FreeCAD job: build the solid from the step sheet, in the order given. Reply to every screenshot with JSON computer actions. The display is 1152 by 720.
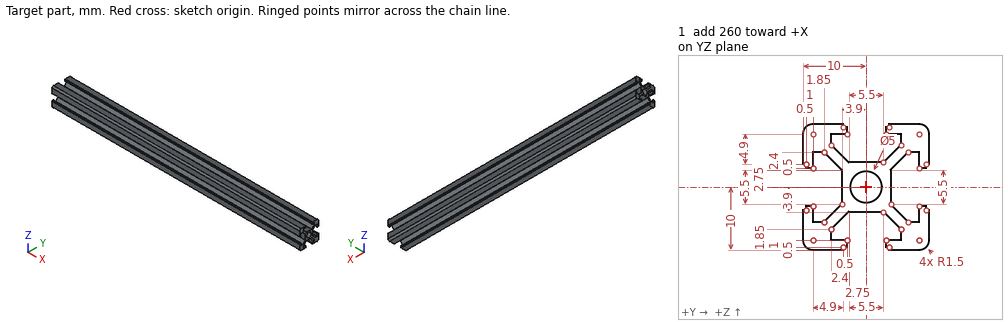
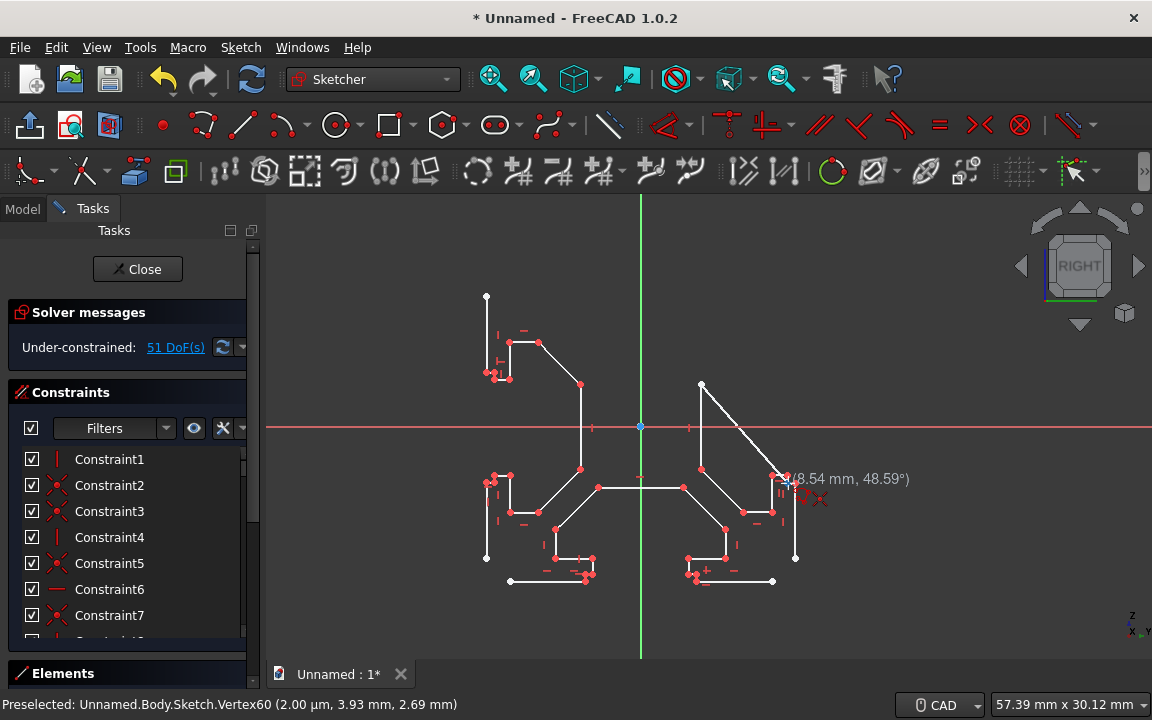
{"action": "left_click", "coordinate": [744, 342]}
{"action": "left_click", "coordinate": [772, 342]}
{"action": "left_click", "coordinate": [772, 379]}
{"action": "left_click", "coordinate": [788, 379]}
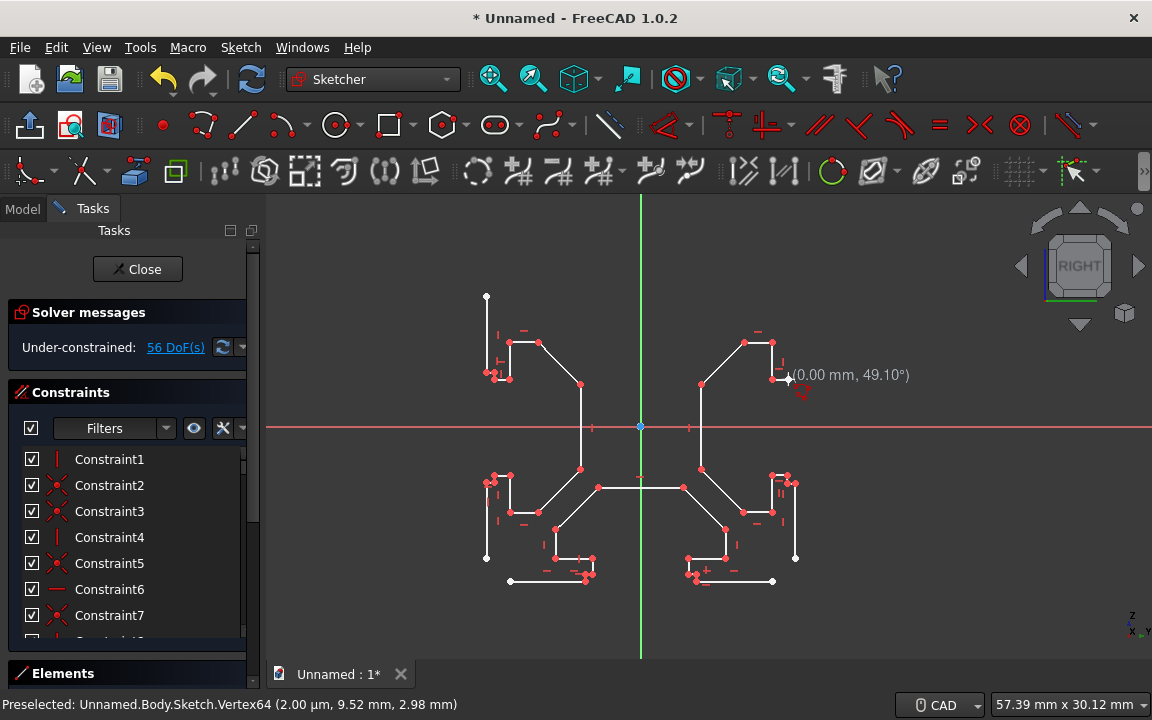
{"action": "scroll", "coordinate": [788, 371], "scroll_direction": "up", "scroll_amount": 4}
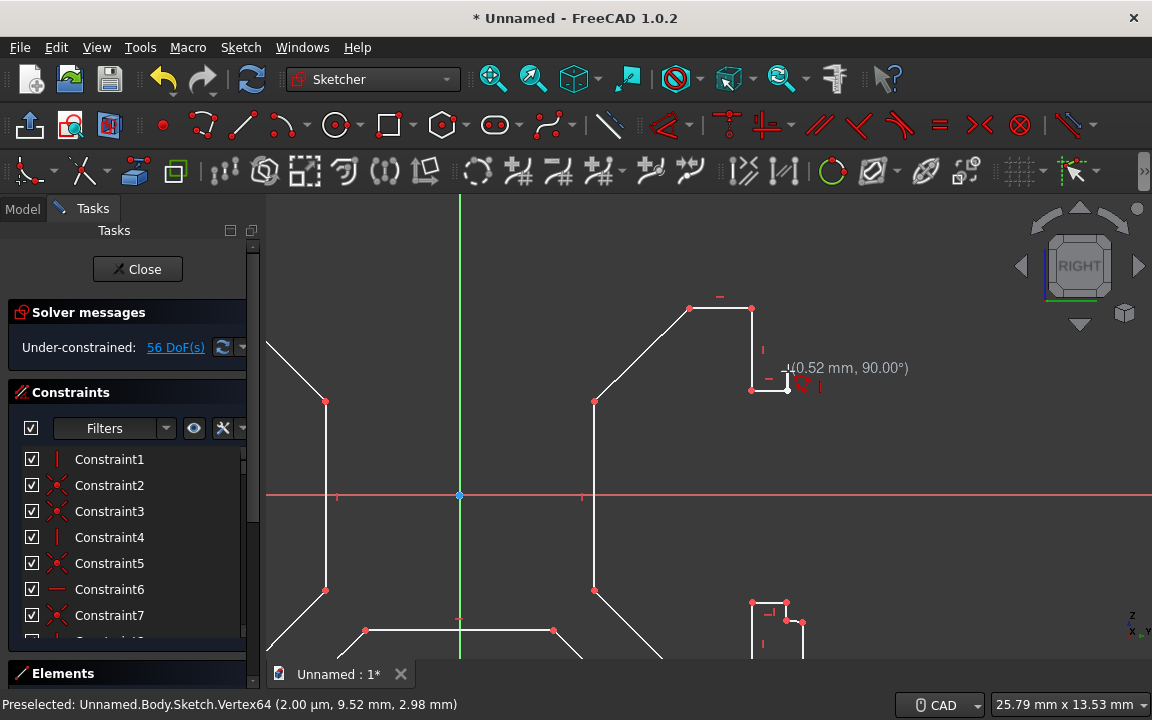
{"action": "left_click", "coordinate": [787, 371]}
{"action": "left_click", "coordinate": [804, 371]}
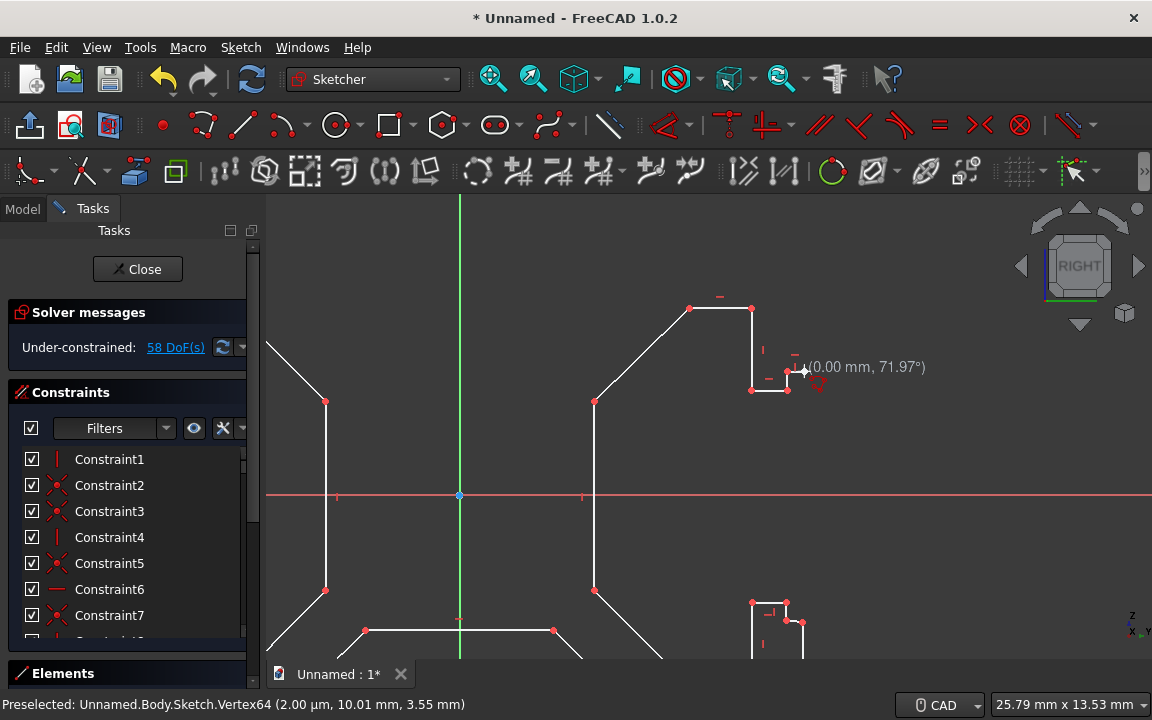
{"action": "scroll", "coordinate": [788, 371], "scroll_direction": "down", "scroll_amount": 4}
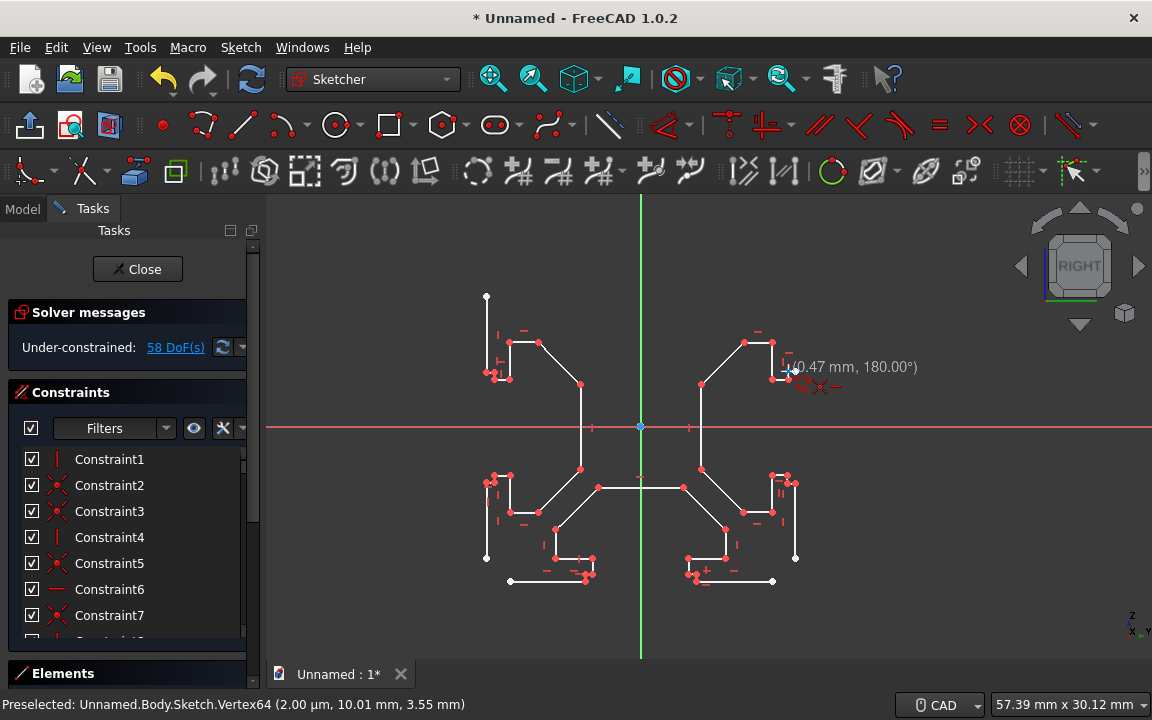
{"action": "left_click", "coordinate": [796, 296]}
{"action": "right_click", "coordinate": [796, 296]}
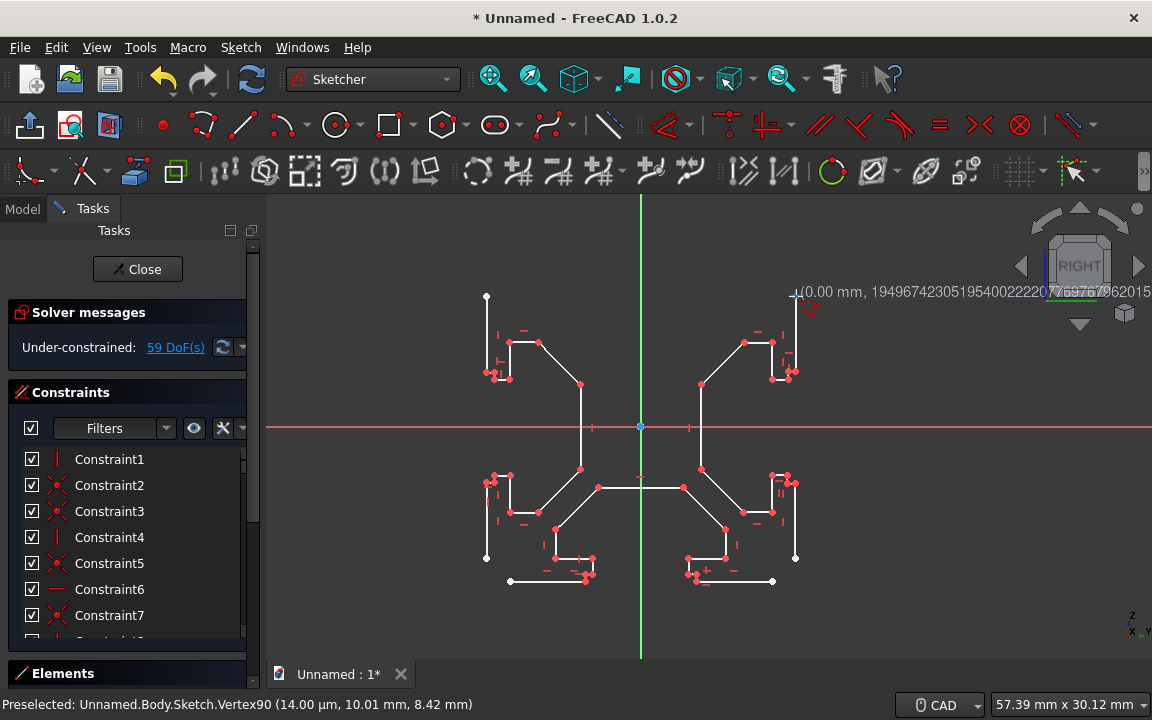
{"action": "left_click", "coordinate": [772, 273]}
{"action": "left_click", "coordinate": [696, 273]}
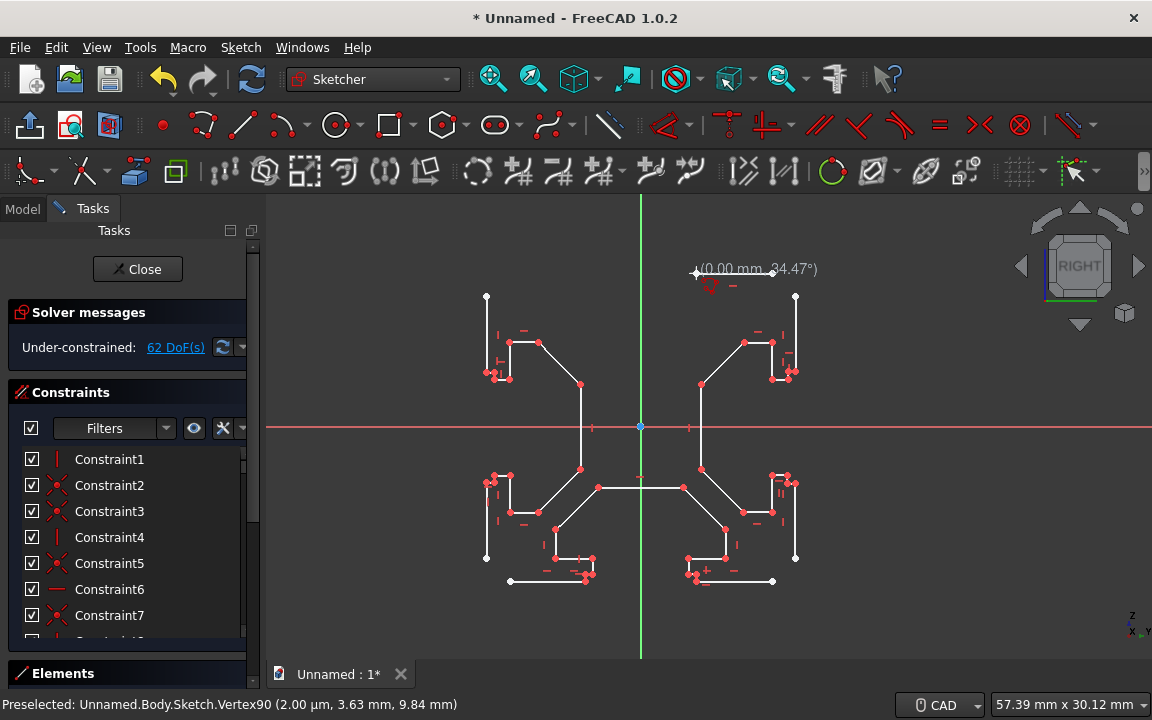
{"action": "scroll", "coordinate": [696, 280], "scroll_direction": "up", "scroll_amount": 4}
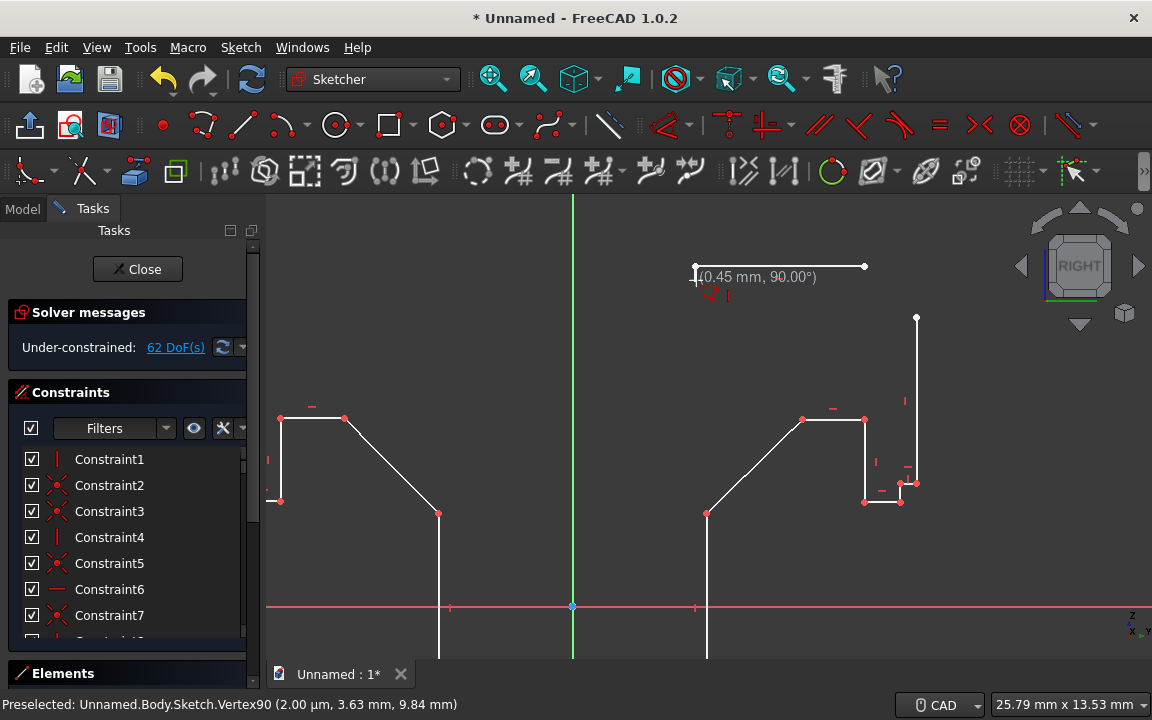
{"action": "left_click", "coordinate": [695, 280]}
{"action": "left_click", "coordinate": [679, 280]}
{"action": "left_click", "coordinate": [679, 315]}
{"action": "left_click", "coordinate": [762, 315]}
{"action": "left_click", "coordinate": [762, 378]}
{"action": "left_click", "coordinate": [667, 473]}
{"action": "left_click", "coordinate": [478, 473]}
{"action": "left_click", "coordinate": [384, 378]}
{"action": "left_click", "coordinate": [384, 315]}
{"action": "left_click", "coordinate": [466, 315]}
{"action": "left_click", "coordinate": [466, 280]}
{"action": "left_click", "coordinate": [449, 280]}
{"action": "left_click", "coordinate": [449, 263]}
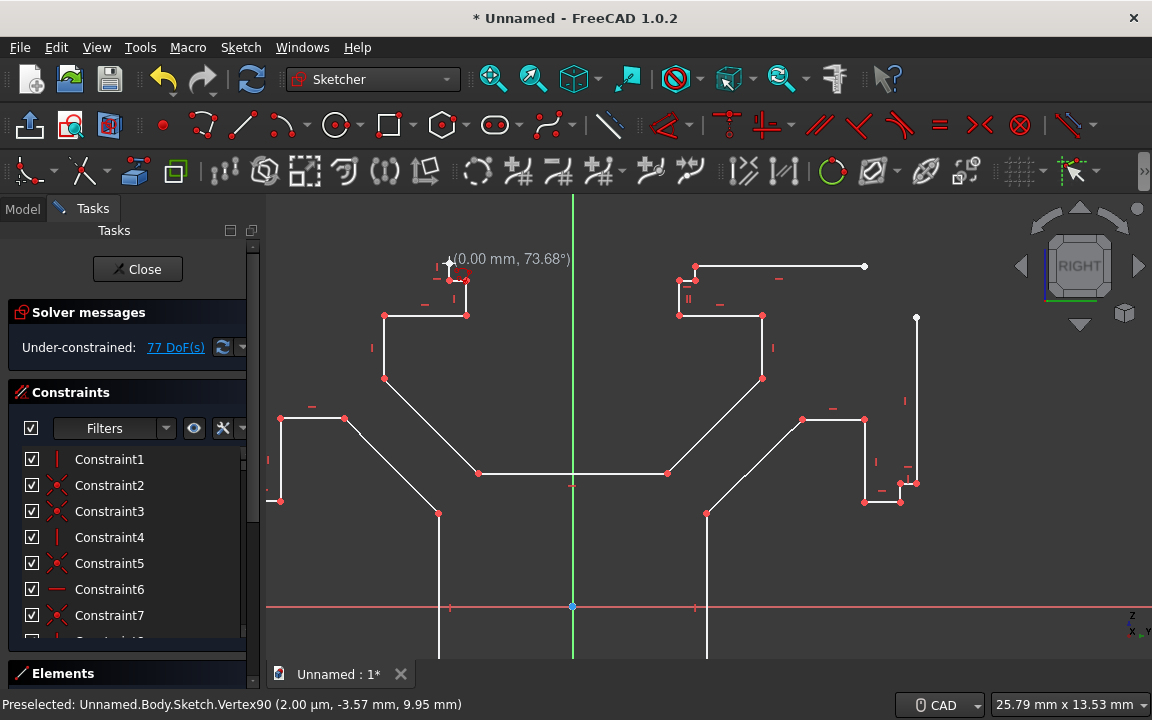
{"action": "scroll", "coordinate": [696, 279], "scroll_direction": "down", "scroll_amount": 4}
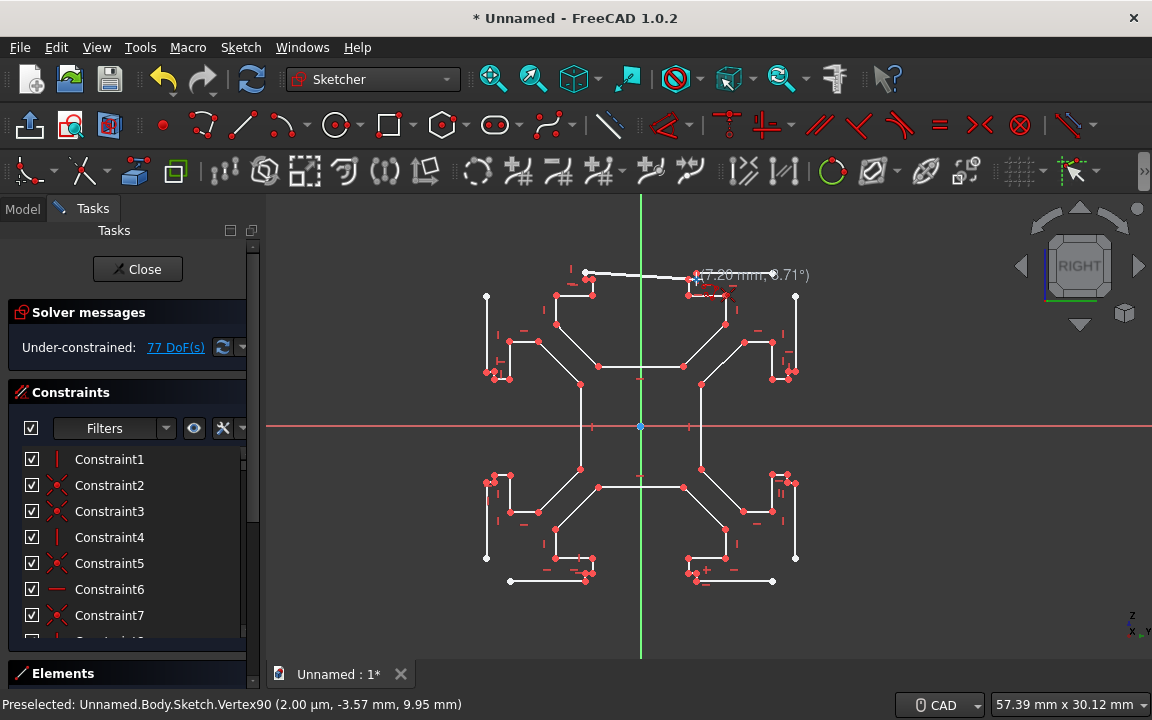
{"action": "left_click", "coordinate": [510, 272]}
{"action": "right_click", "coordinate": [510, 272]}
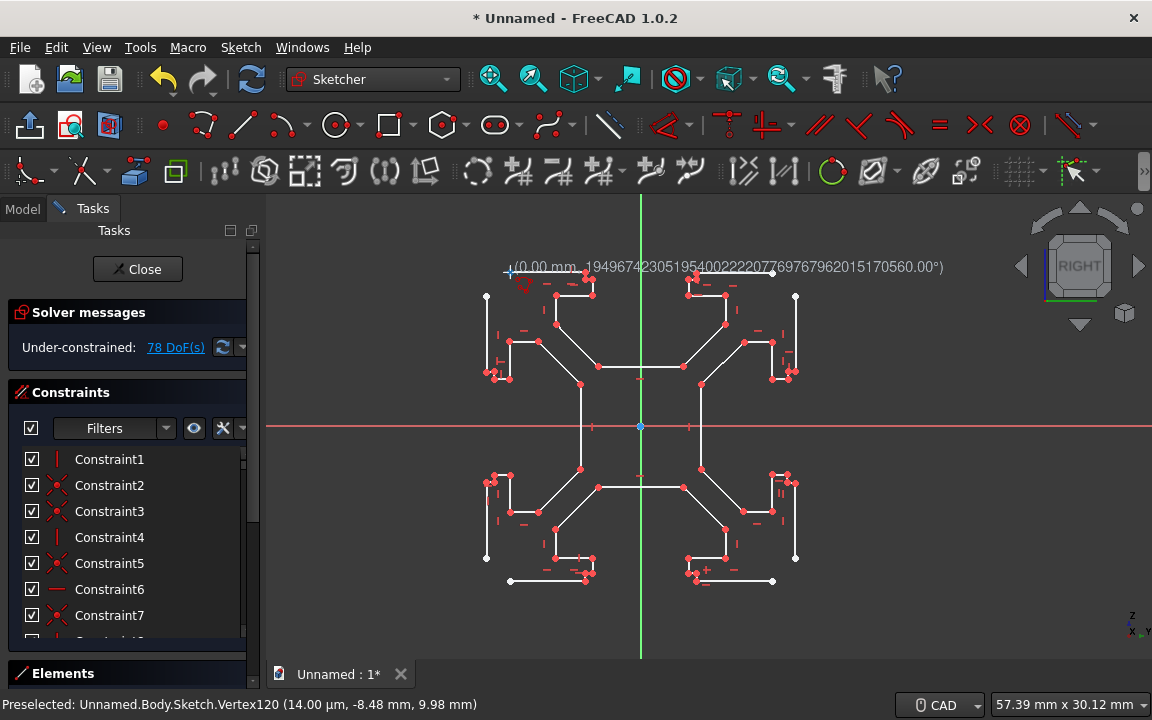
{"action": "left_click", "coordinate": [310, 126]}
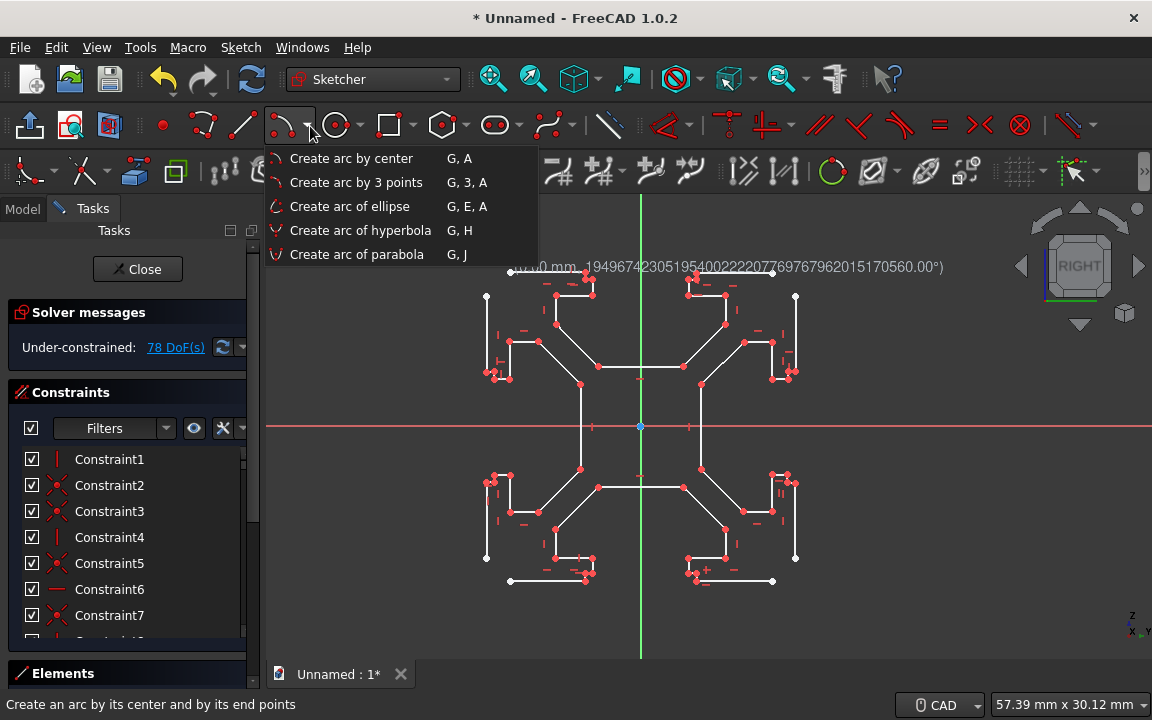
{"action": "left_click", "coordinate": [402, 182]}